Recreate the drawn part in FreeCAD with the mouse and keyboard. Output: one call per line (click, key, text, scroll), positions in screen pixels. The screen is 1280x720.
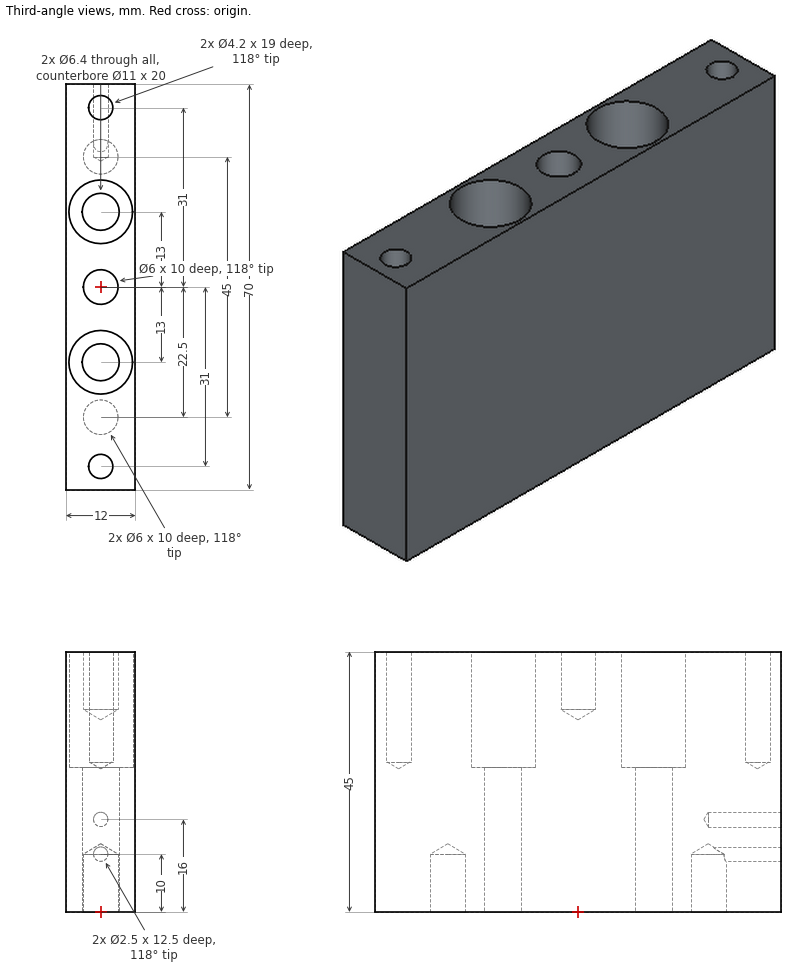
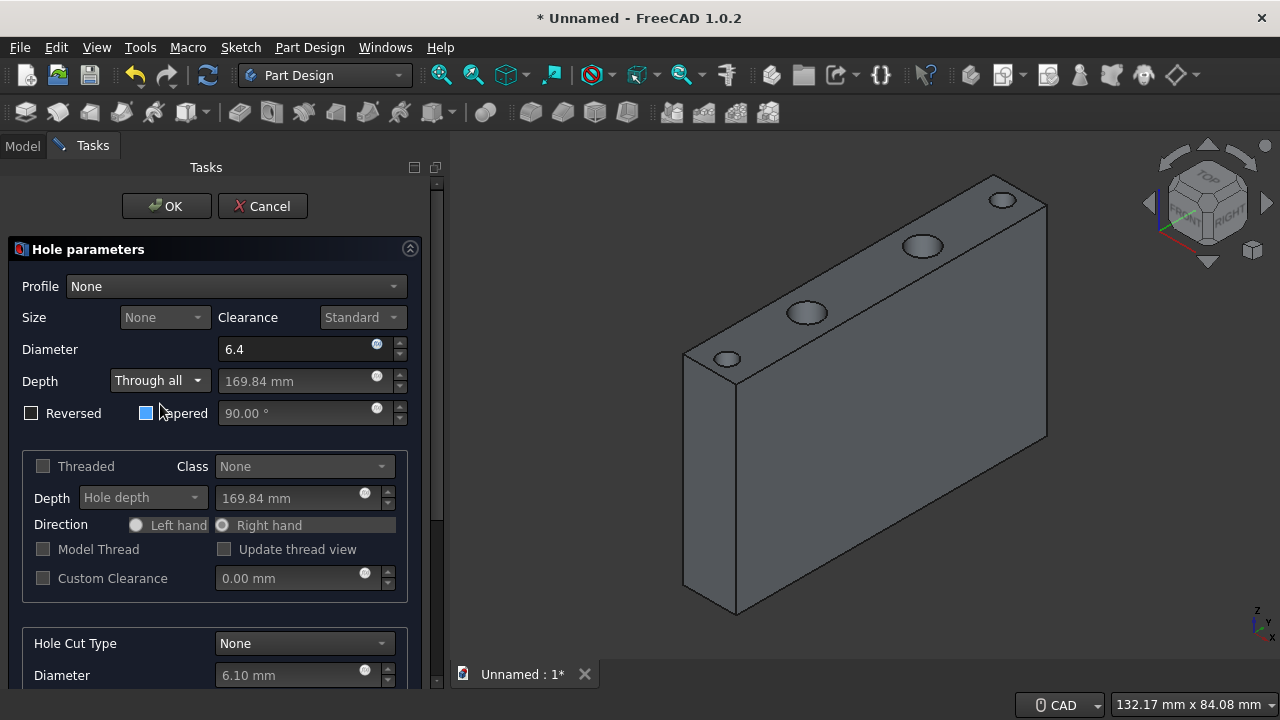
click(306, 644)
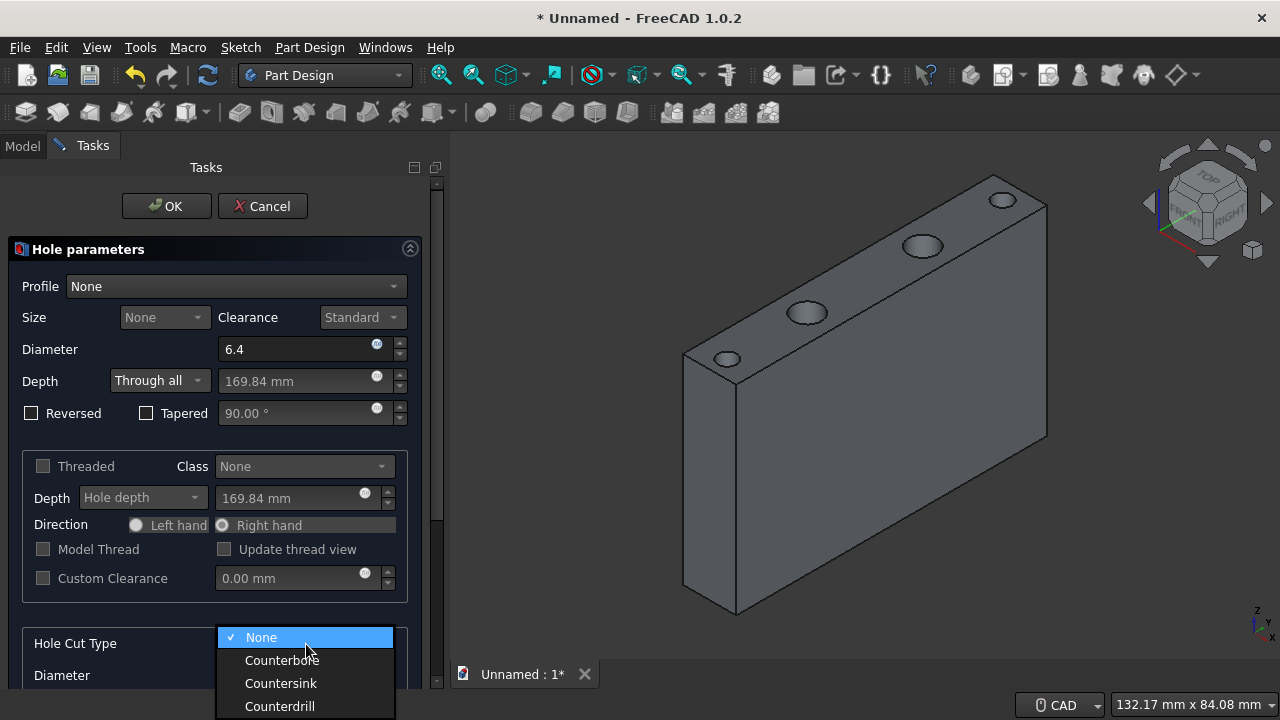
click(304, 660)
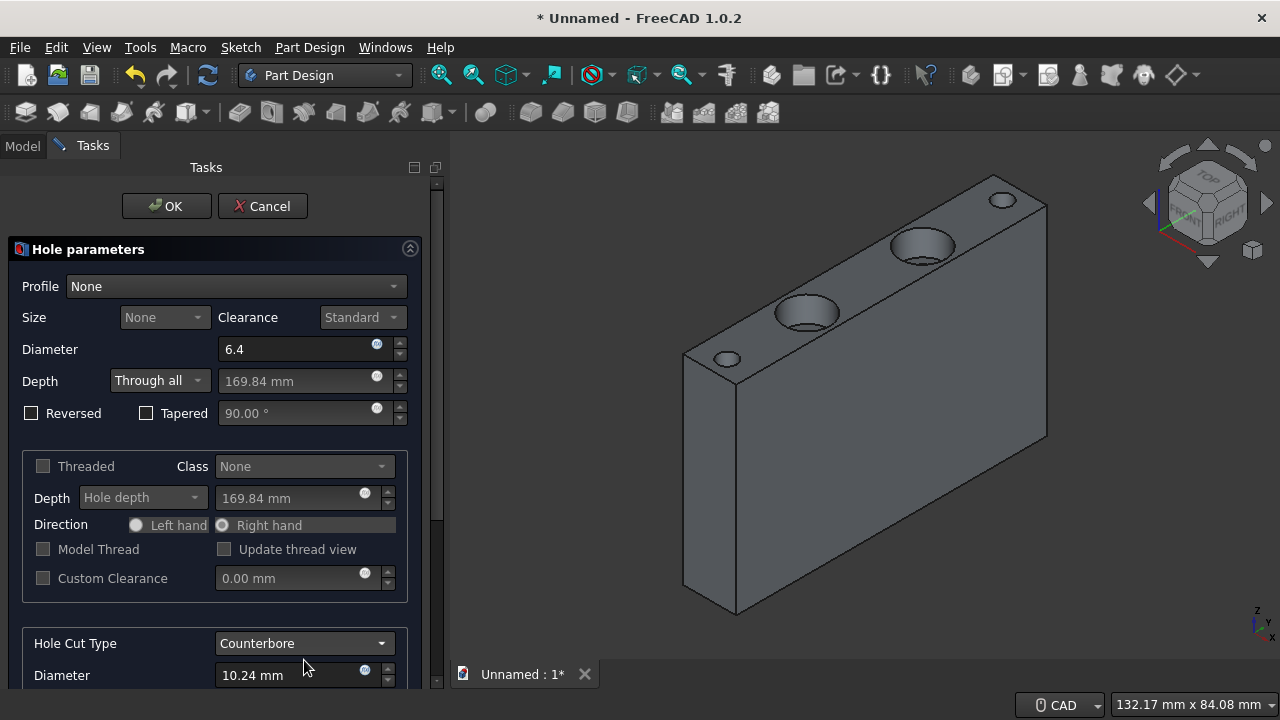
triple_click(298, 675)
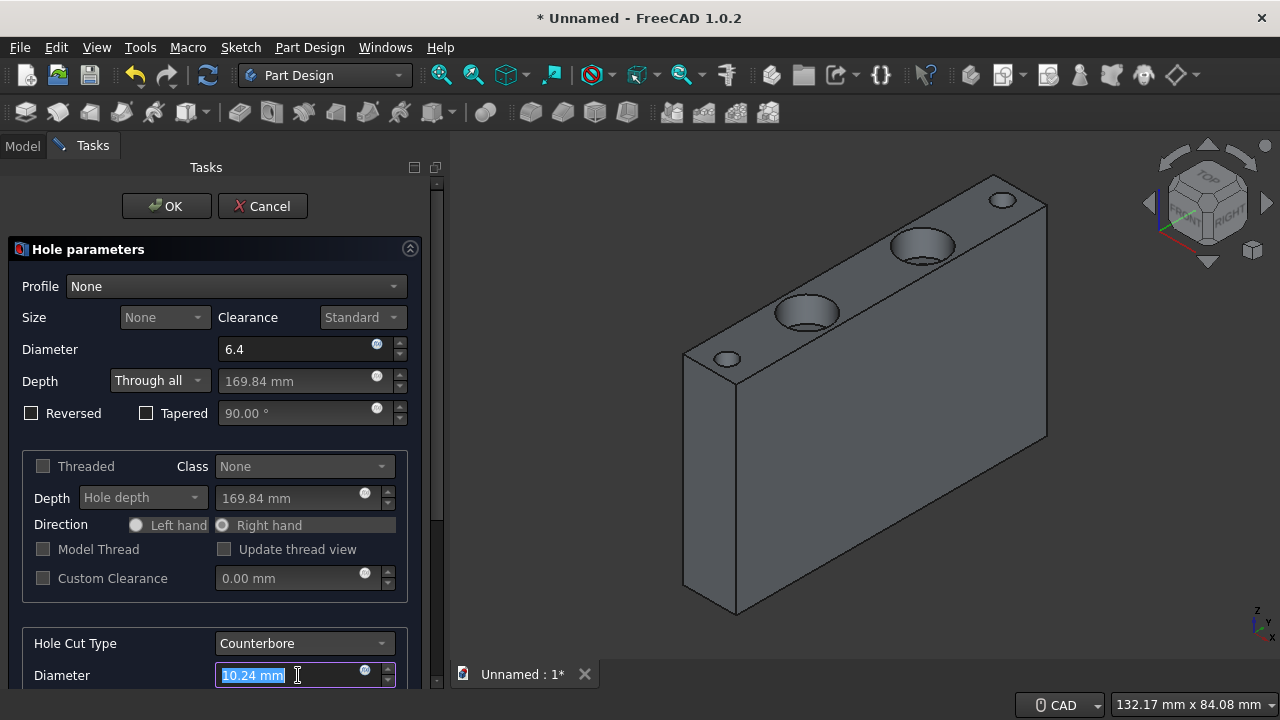
text(11)
key(Tab)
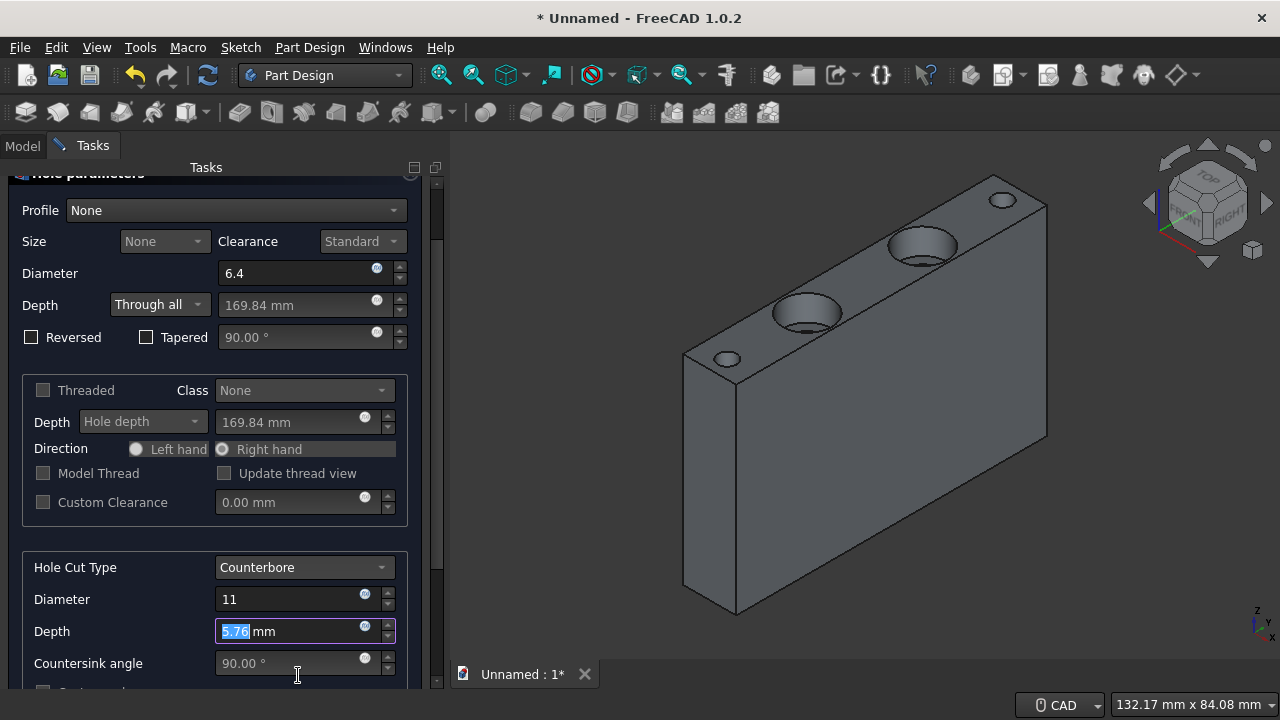
text(20)
key(Tab)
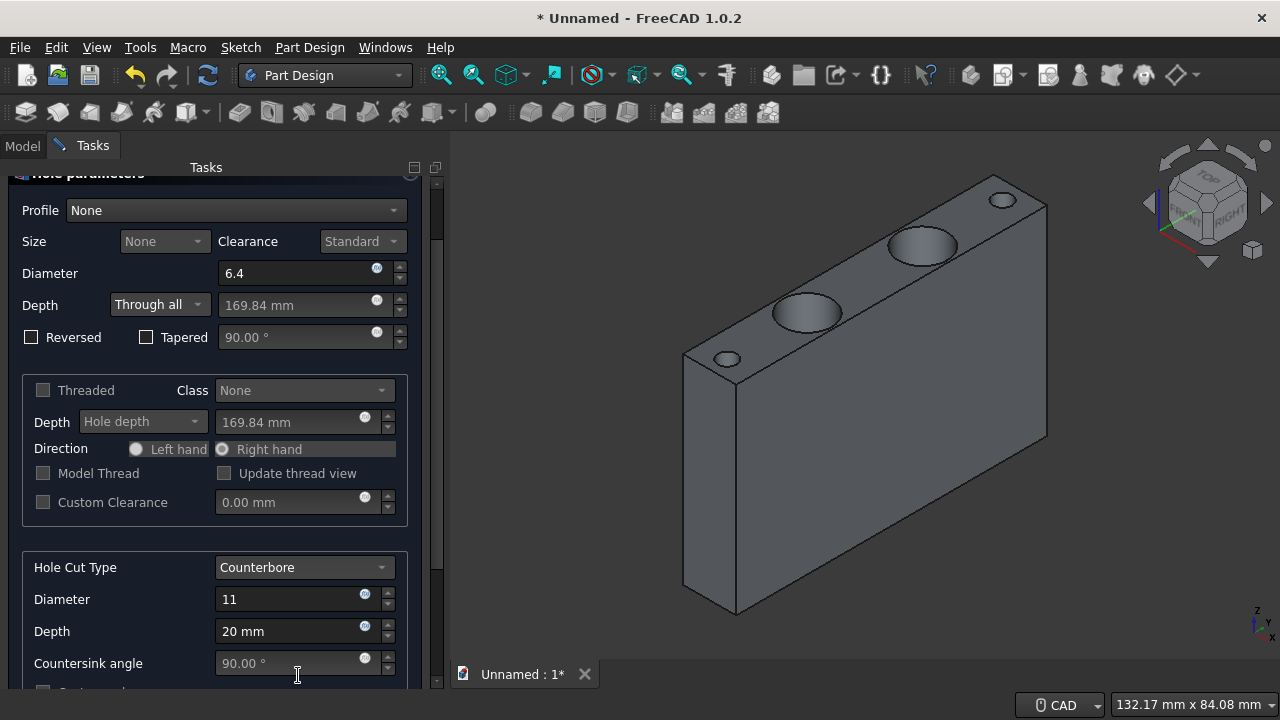
scroll(437, 432, up, 3)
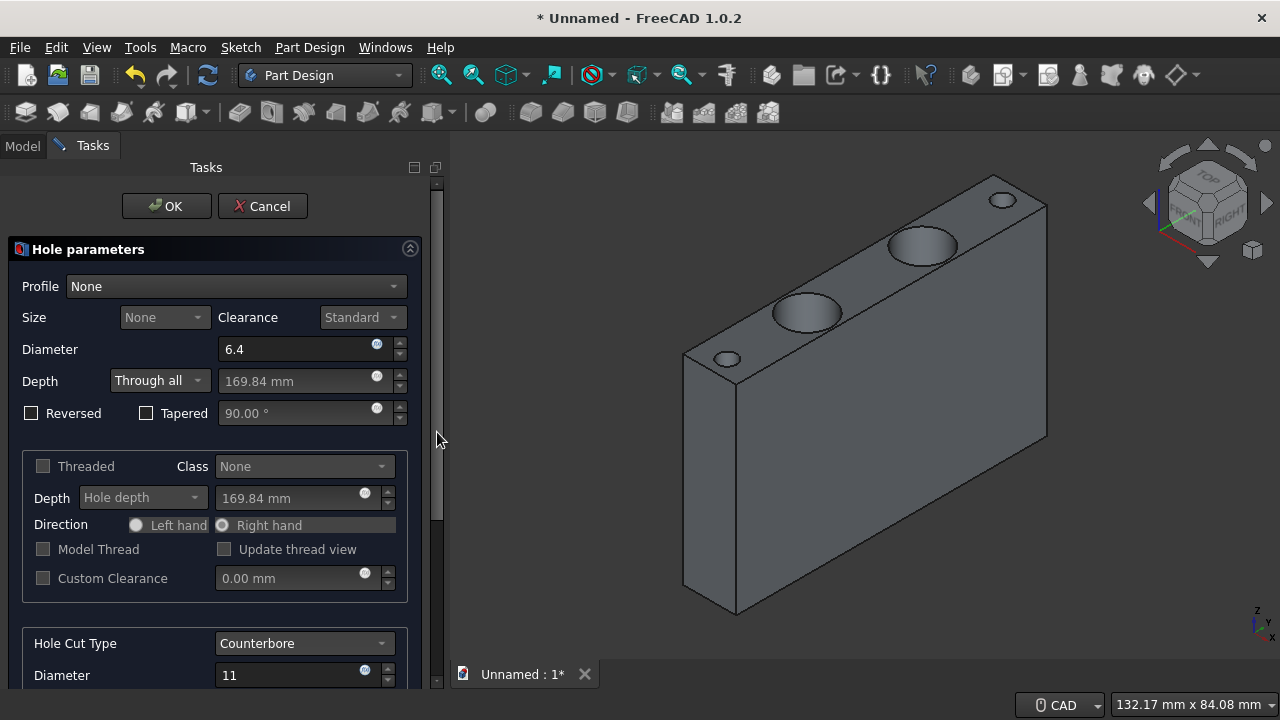
click(167, 206)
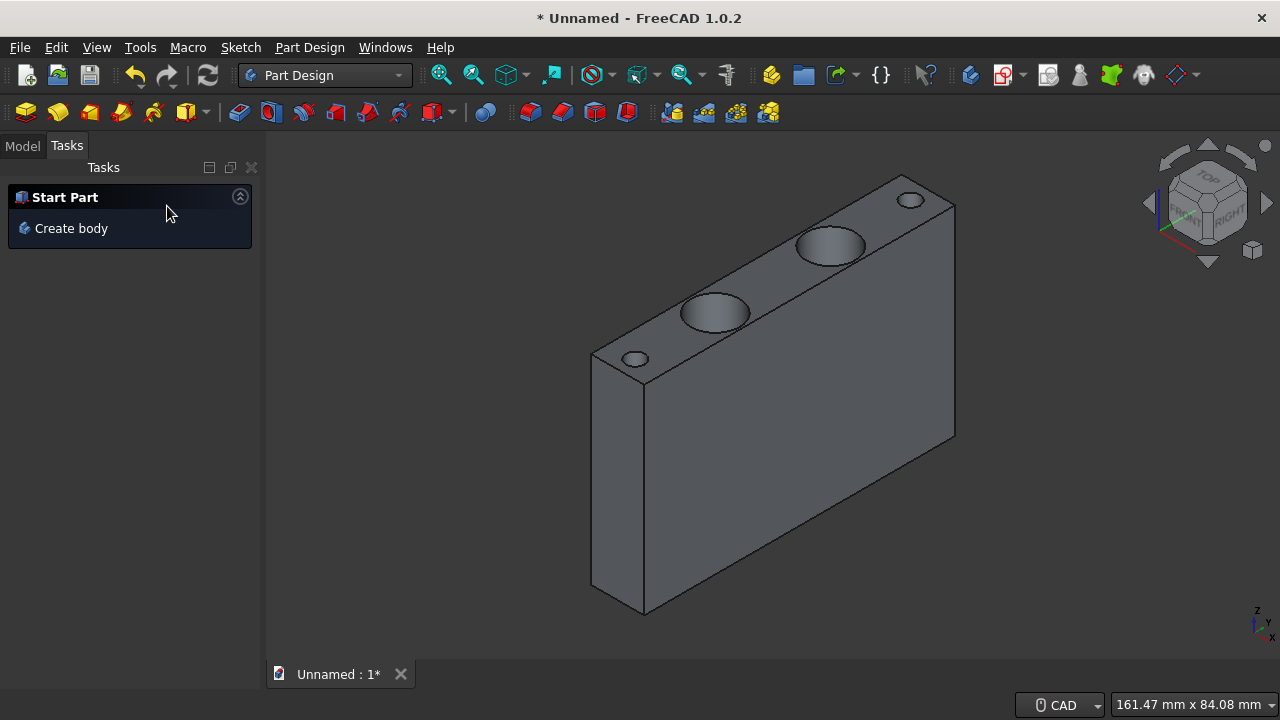
click(773, 279)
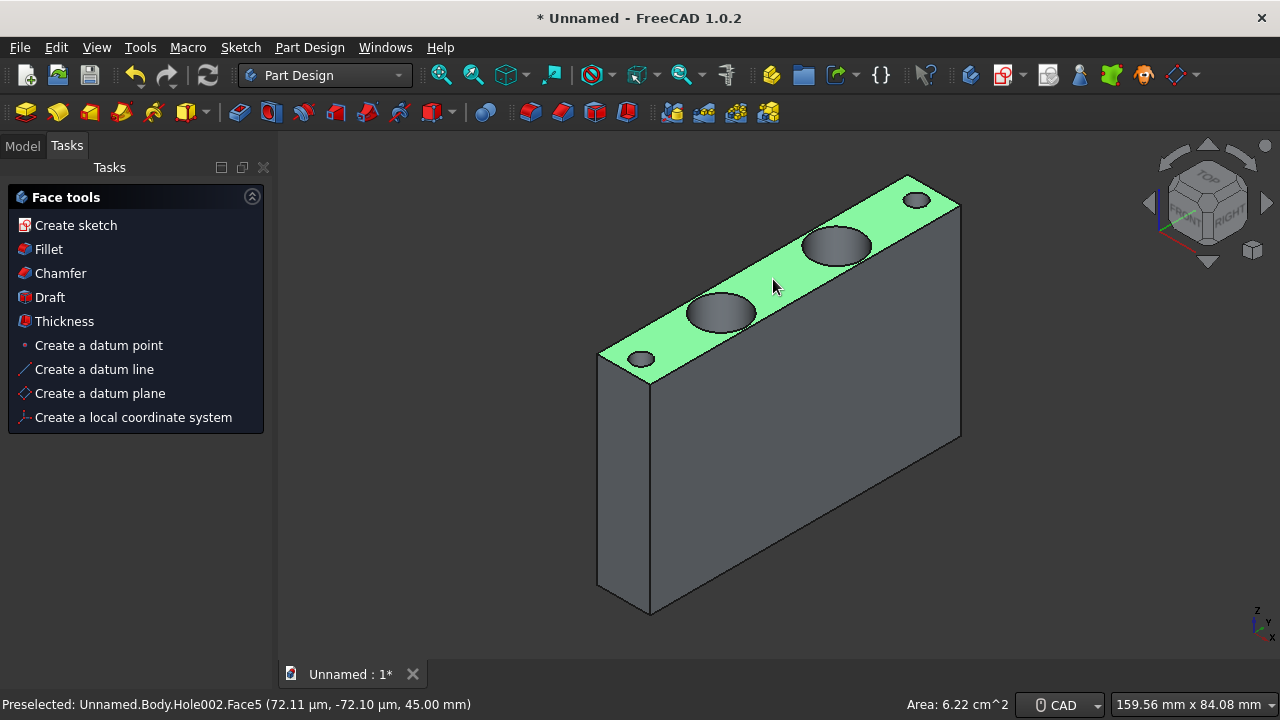
click(1004, 76)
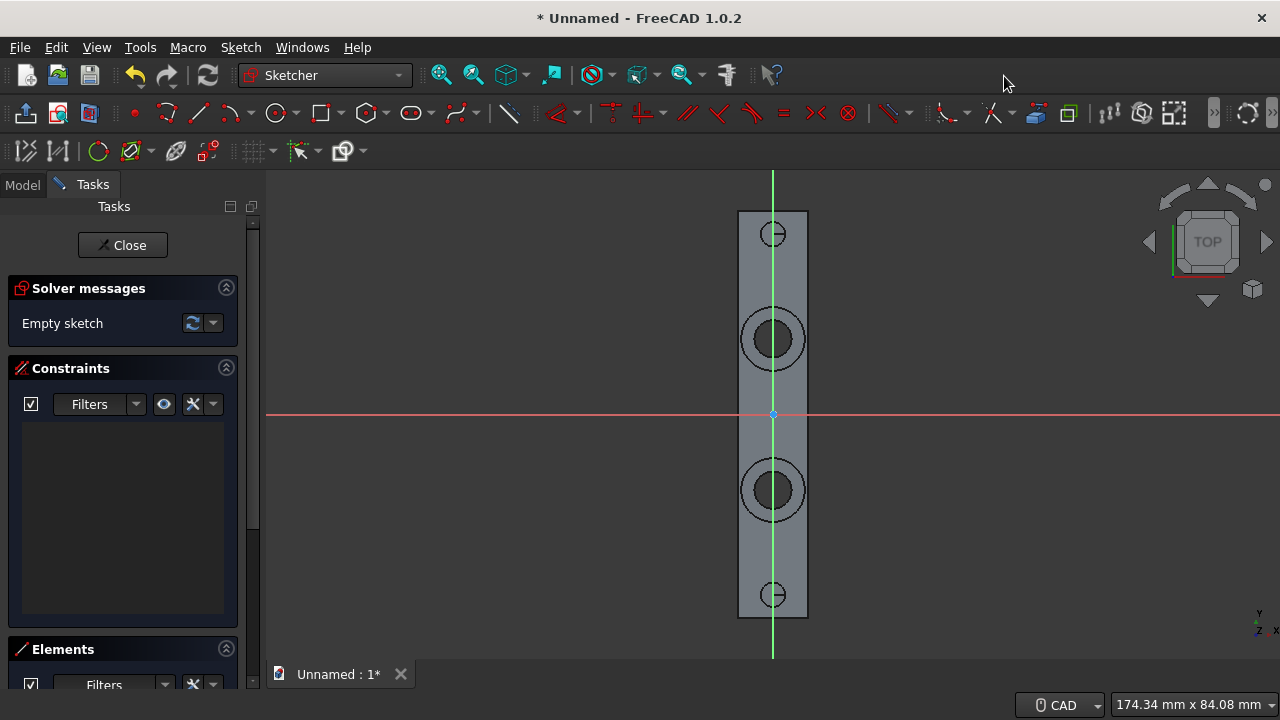
scroll(782, 414, up, 11)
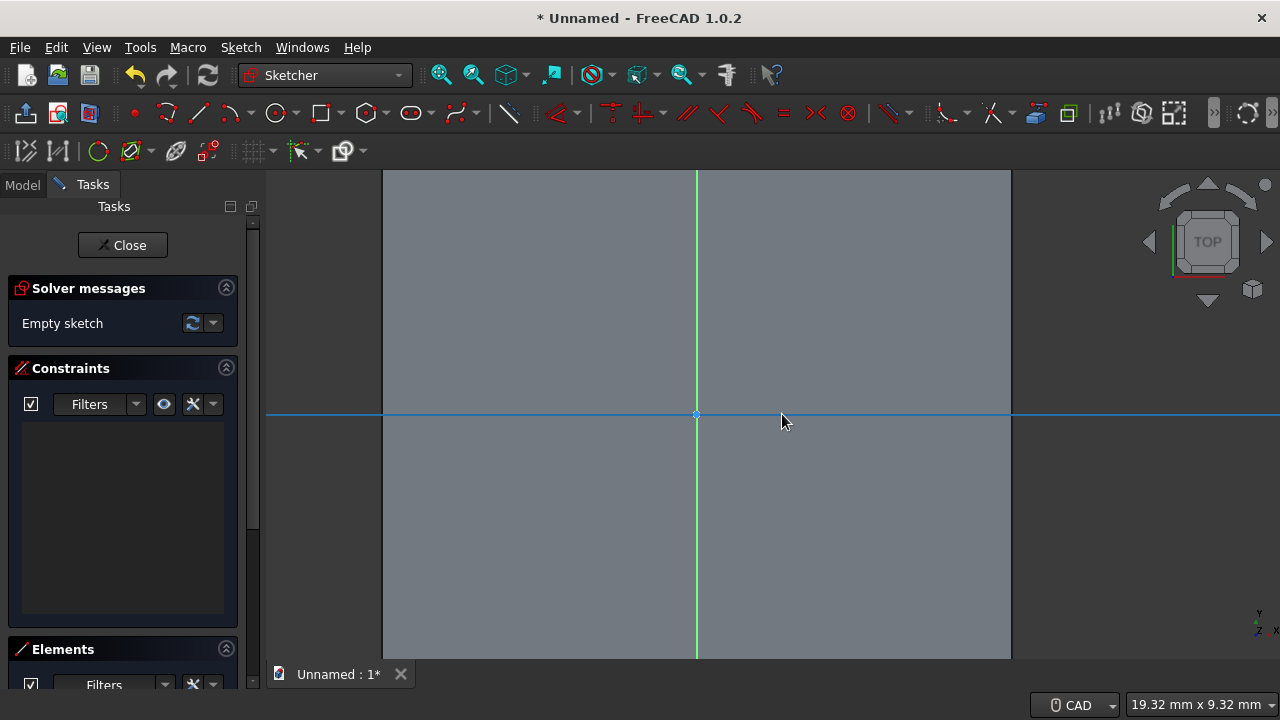
click(276, 114)